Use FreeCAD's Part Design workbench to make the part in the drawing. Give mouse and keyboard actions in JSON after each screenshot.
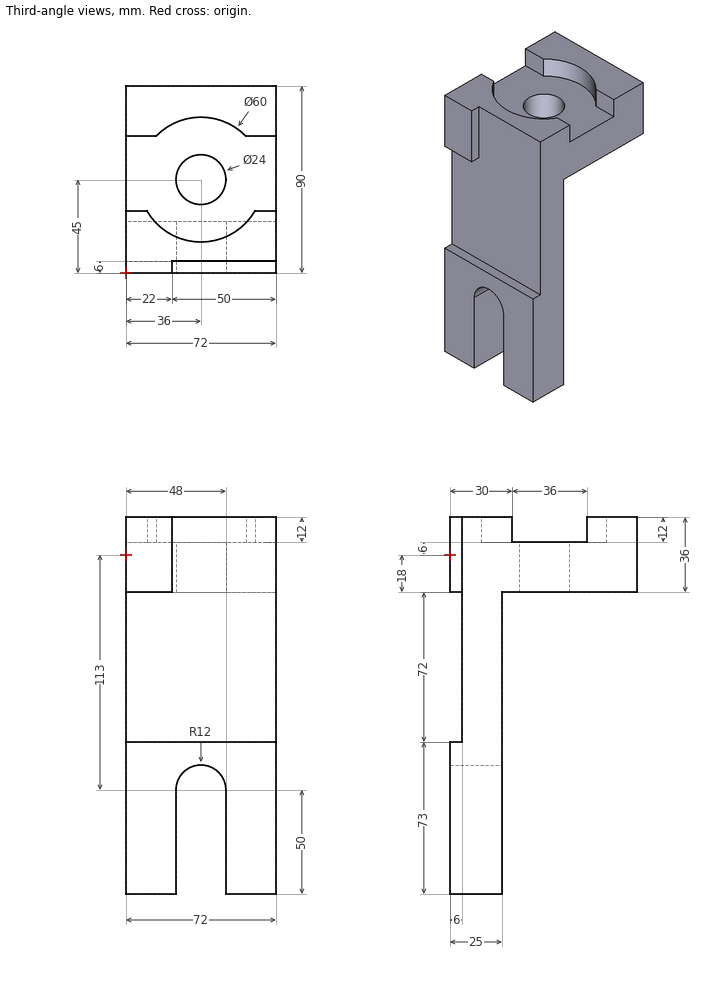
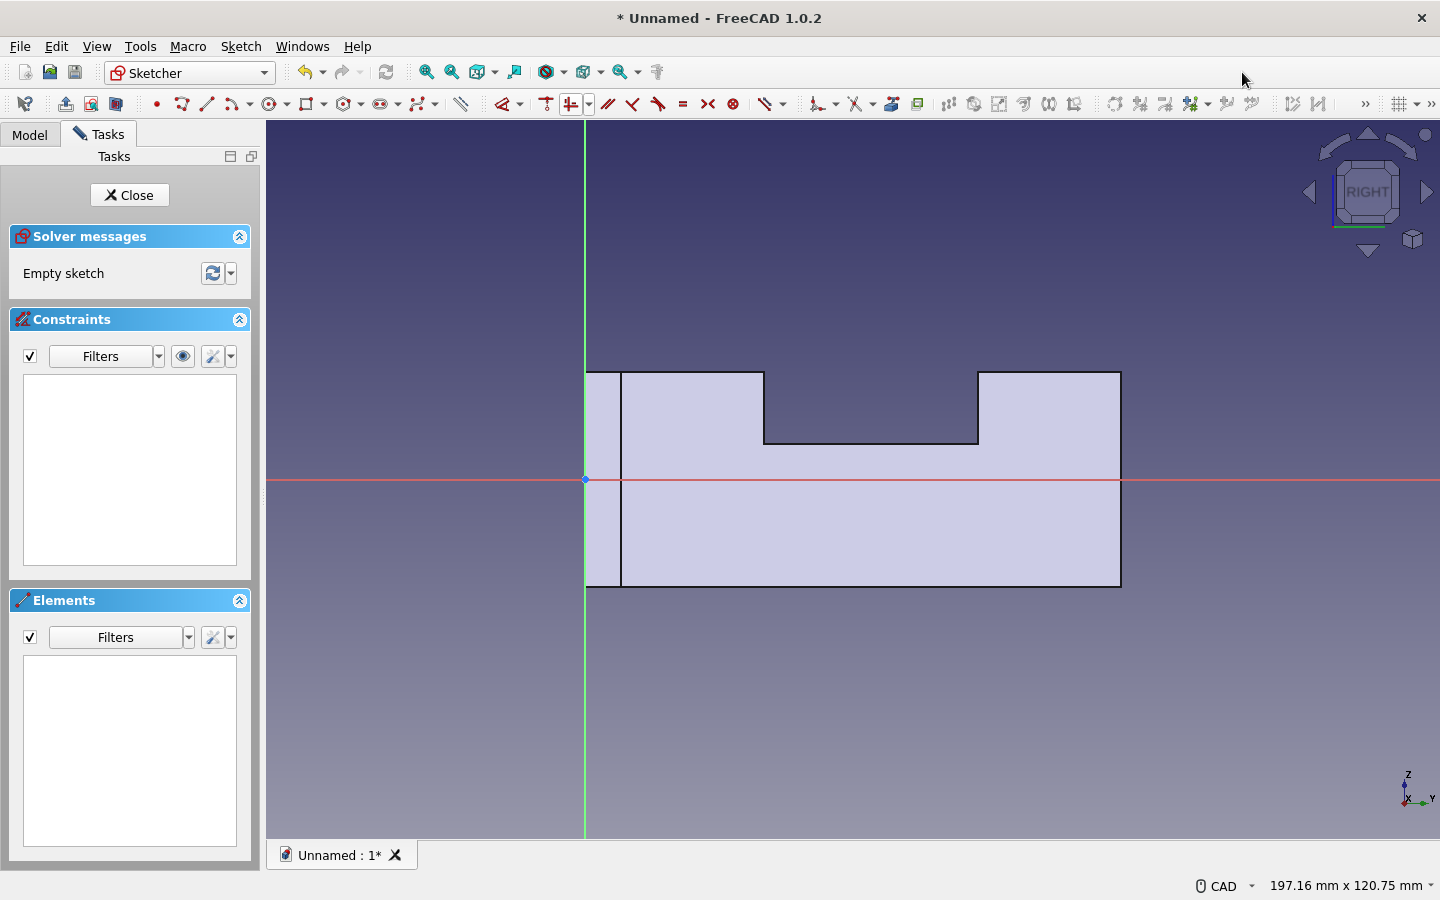
{"action": "scroll", "coordinate": [887, 148], "scroll_direction": "down", "scroll_amount": 4}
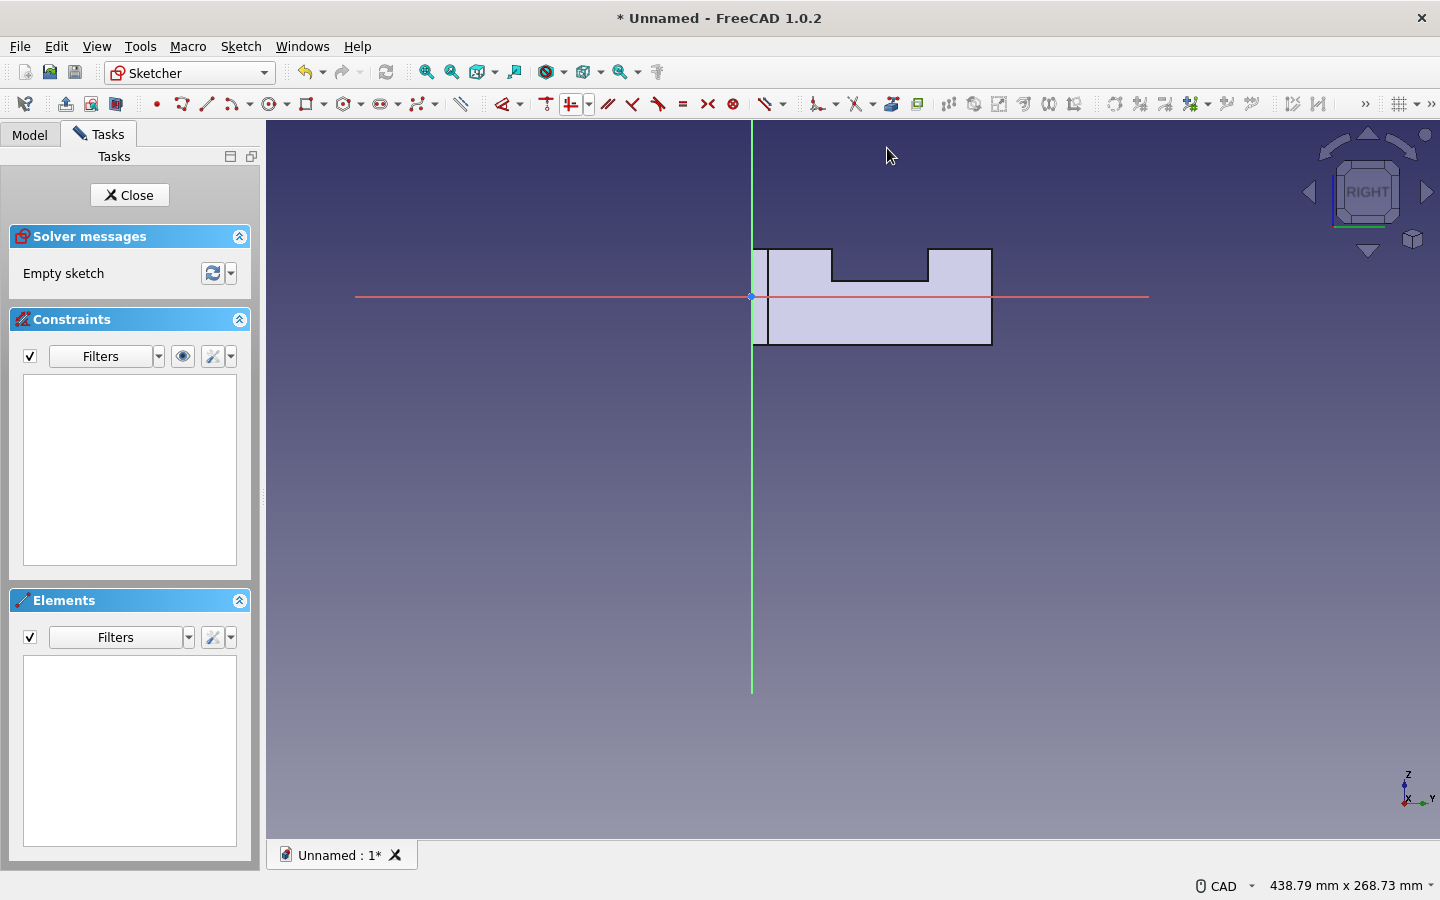
{"action": "key", "text": "g m"}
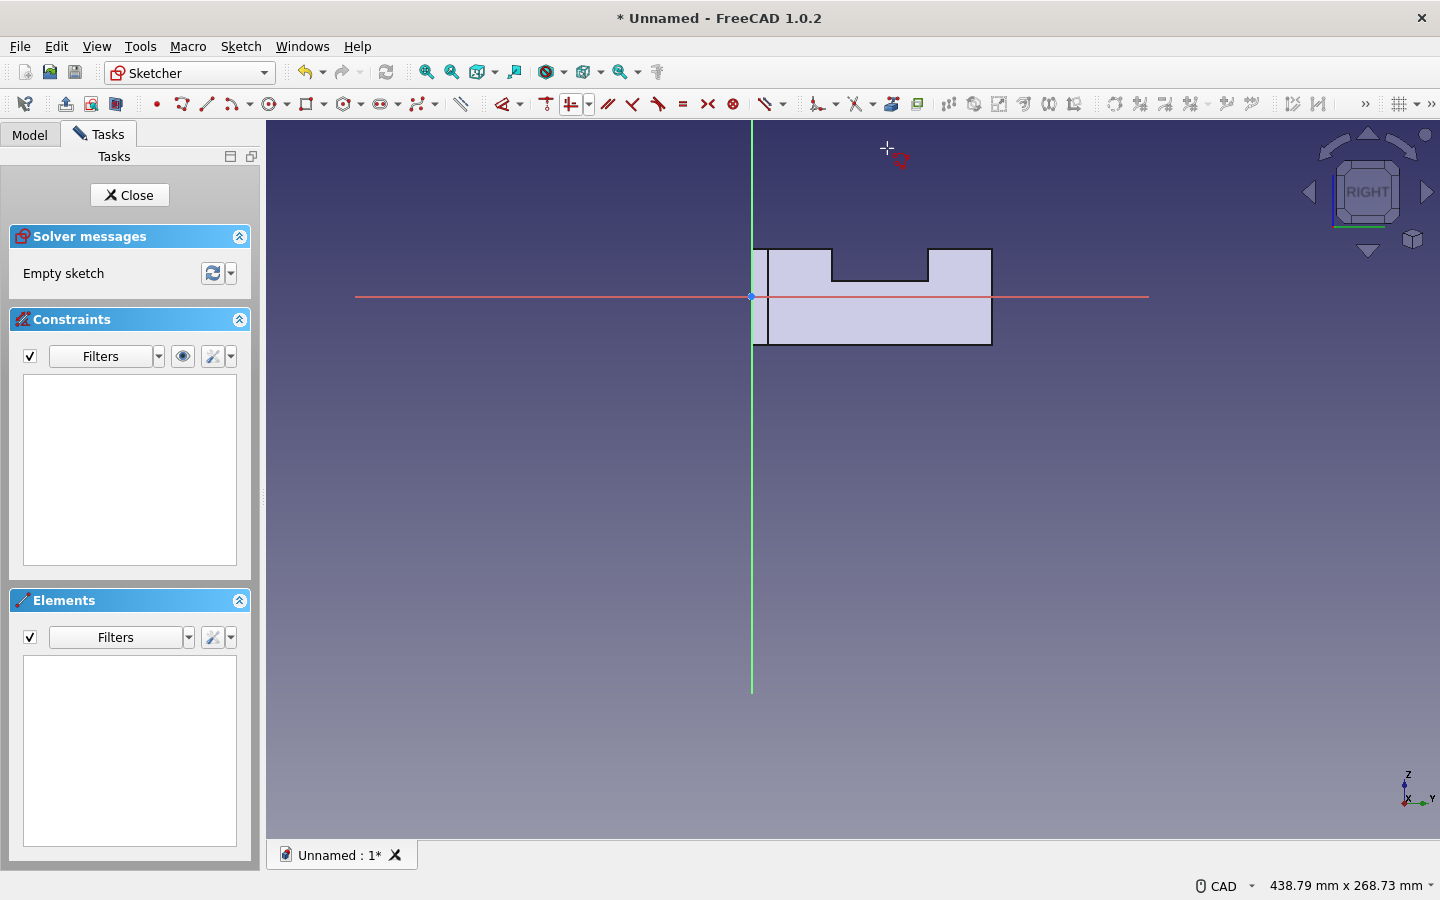
{"action": "left_click", "coordinate": [768, 345]}
{"action": "left_click", "coordinate": [768, 538]}
{"action": "left_click", "coordinate": [752, 538]}
{"action": "left_click", "coordinate": [761, 733]}
{"action": "left_click", "coordinate": [819, 733]}
{"action": "left_click", "coordinate": [819, 345]}
{"action": "left_click", "coordinate": [768, 346]}
{"action": "key", "text": "Escape"}
{"action": "key", "text": "Escape"}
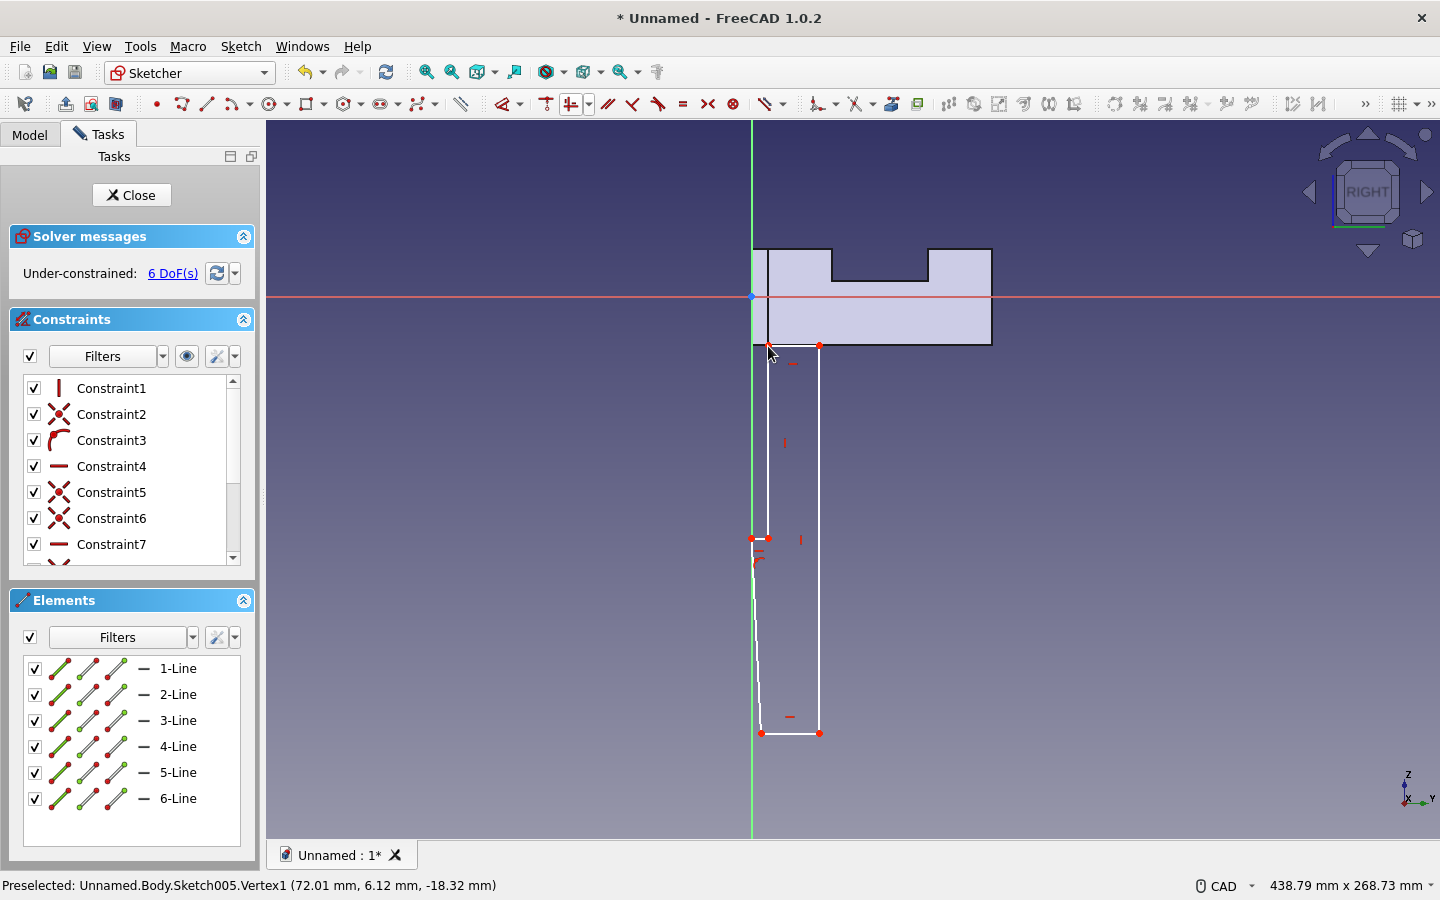
{"action": "left_click", "coordinate": [754, 598]}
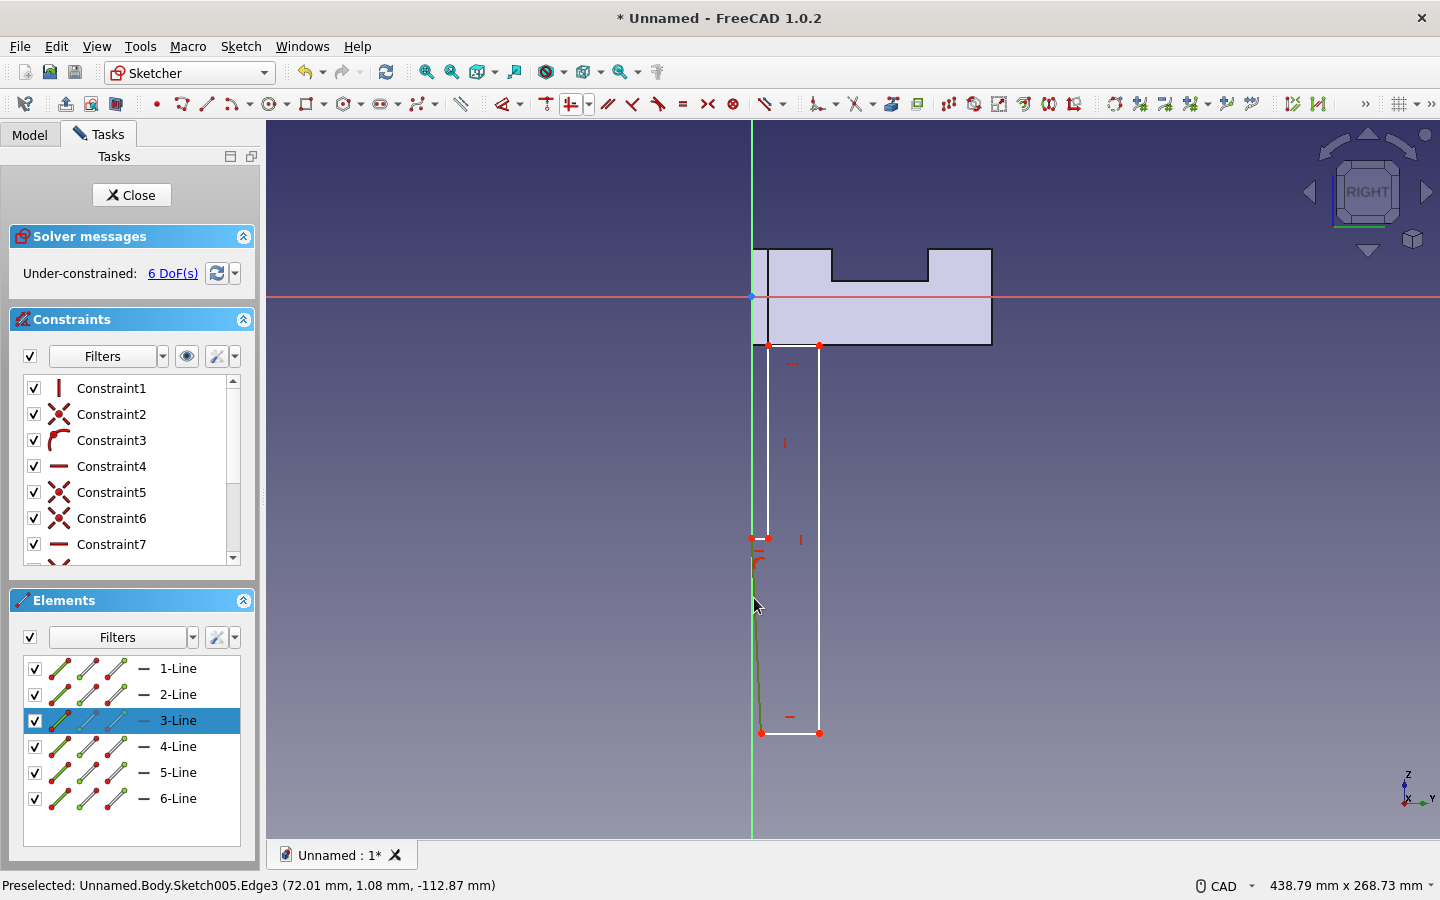
{"action": "key", "text": "v"}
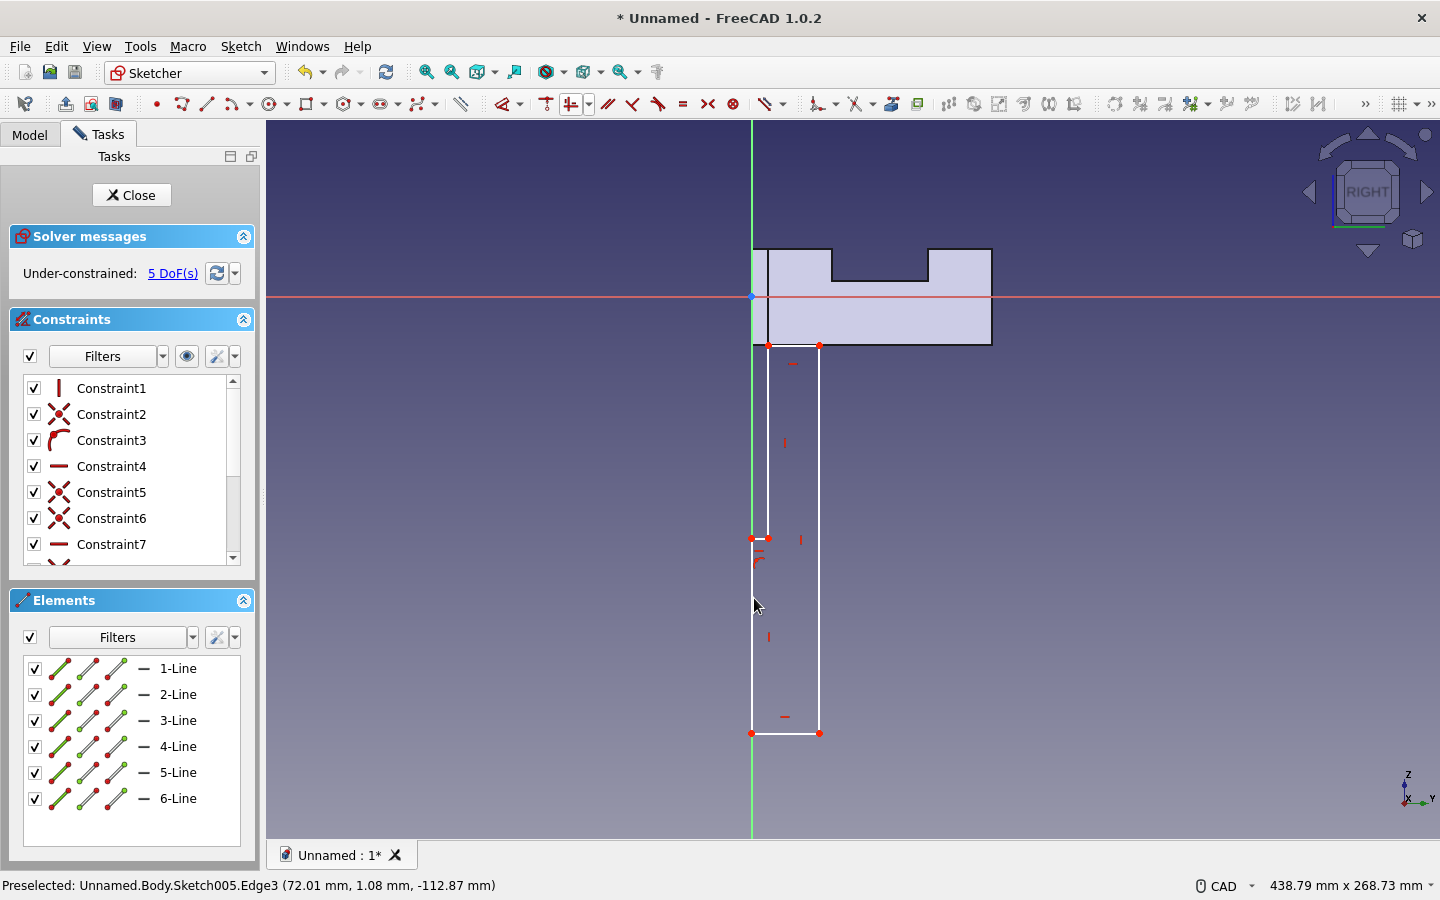
{"action": "key", "text": "d"}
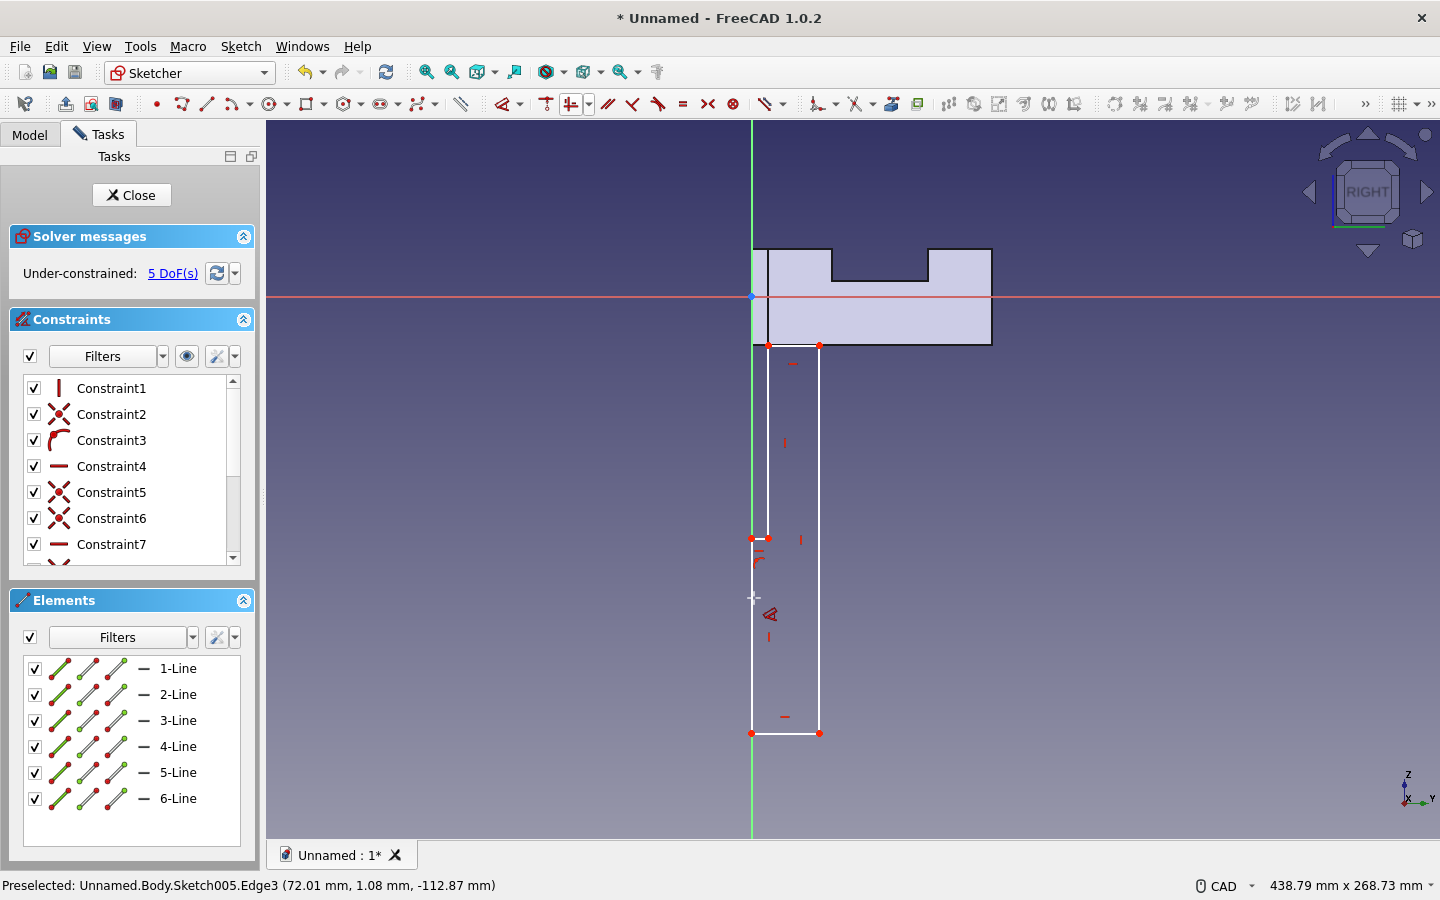
{"action": "scroll", "coordinate": [760, 539], "scroll_direction": "up", "scroll_amount": 5}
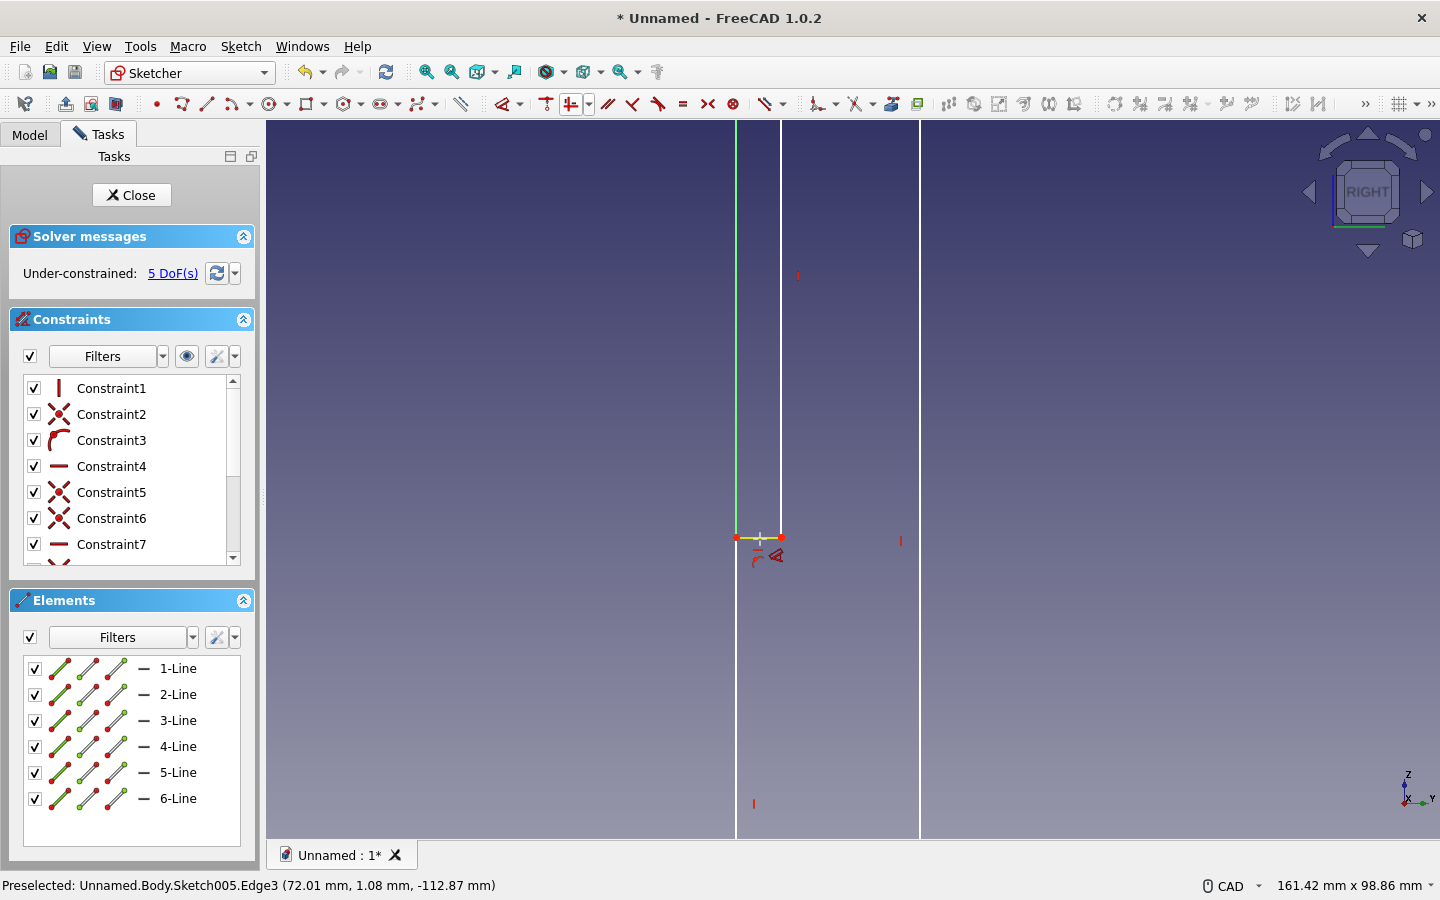
{"action": "left_click", "coordinate": [759, 538]}
{"action": "left_click", "coordinate": [759, 572]}